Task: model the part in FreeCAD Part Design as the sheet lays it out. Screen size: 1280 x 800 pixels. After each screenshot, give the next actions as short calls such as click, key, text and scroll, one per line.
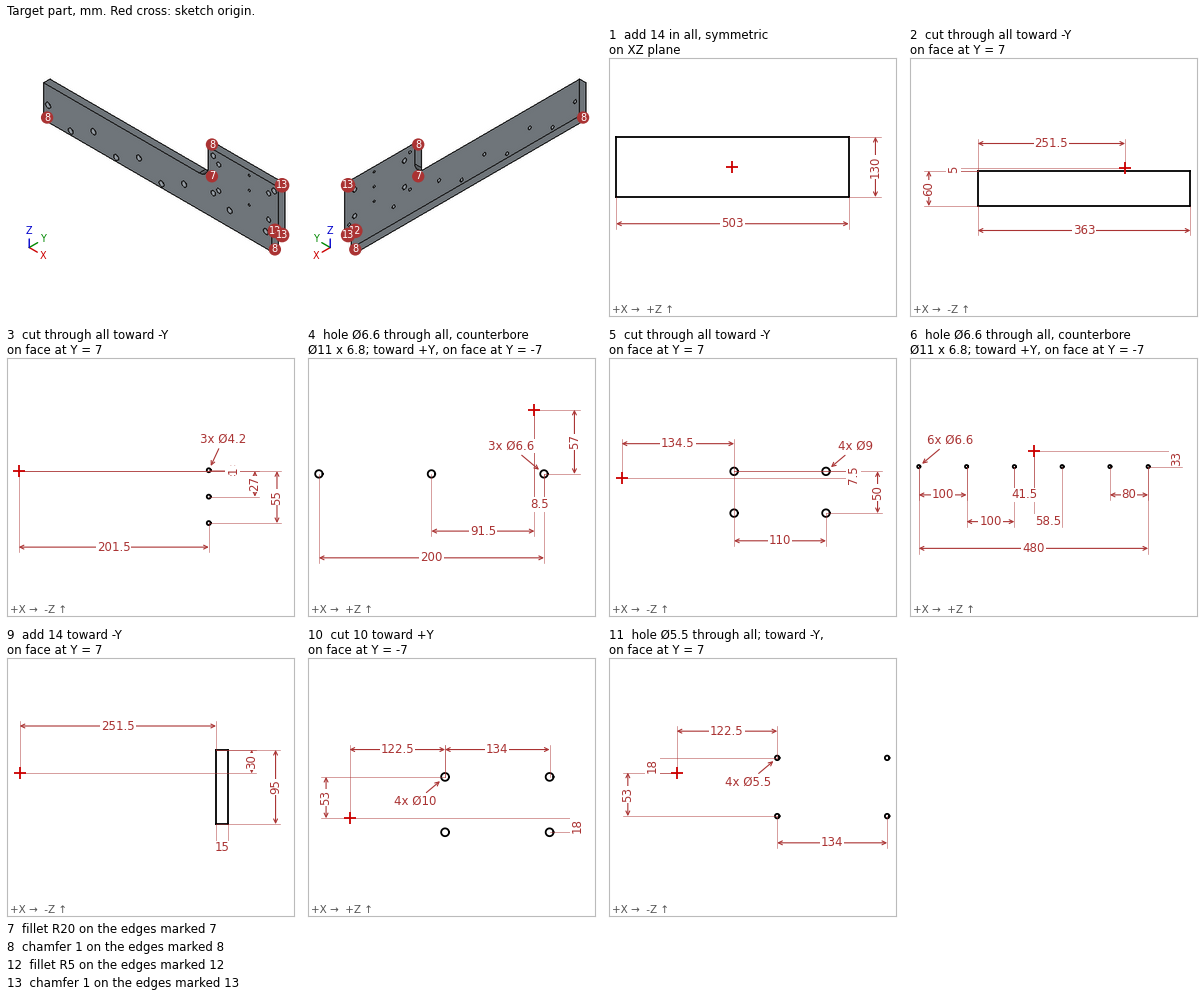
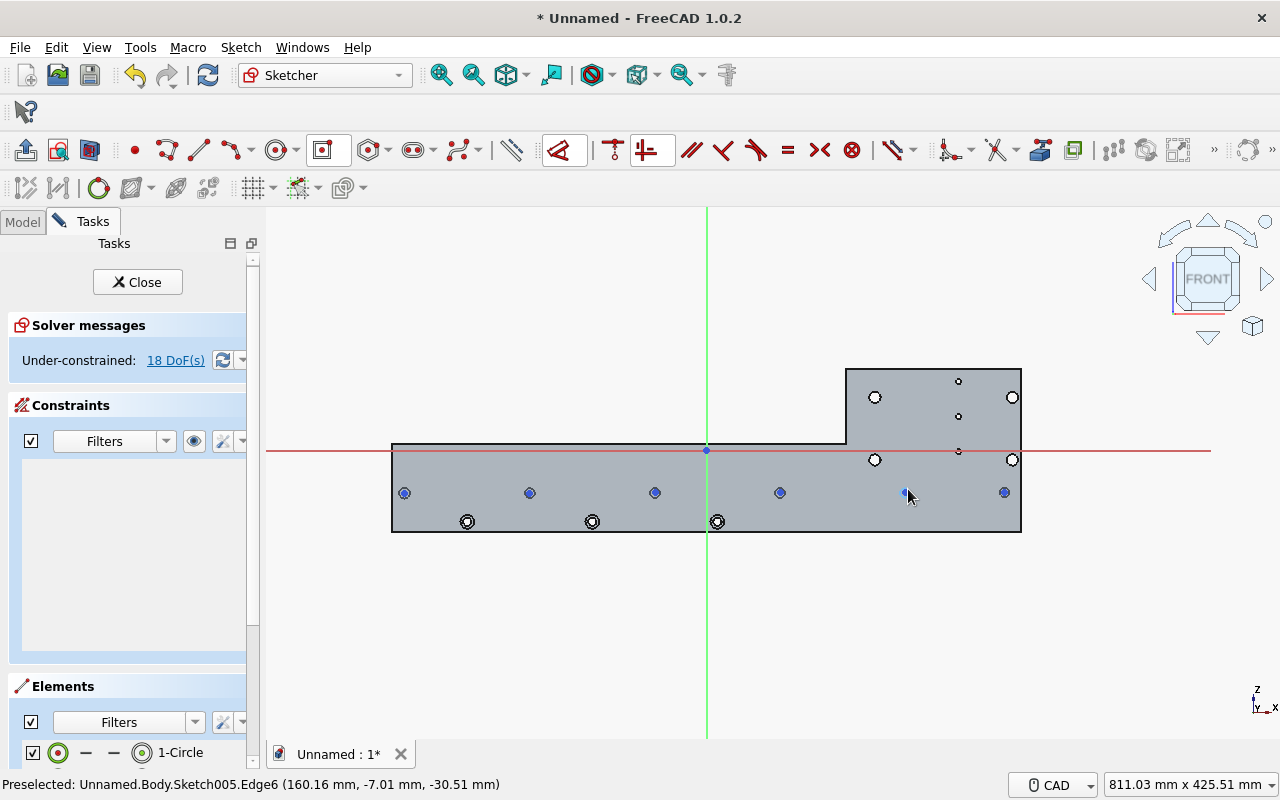
scroll(1008, 489, up, 6)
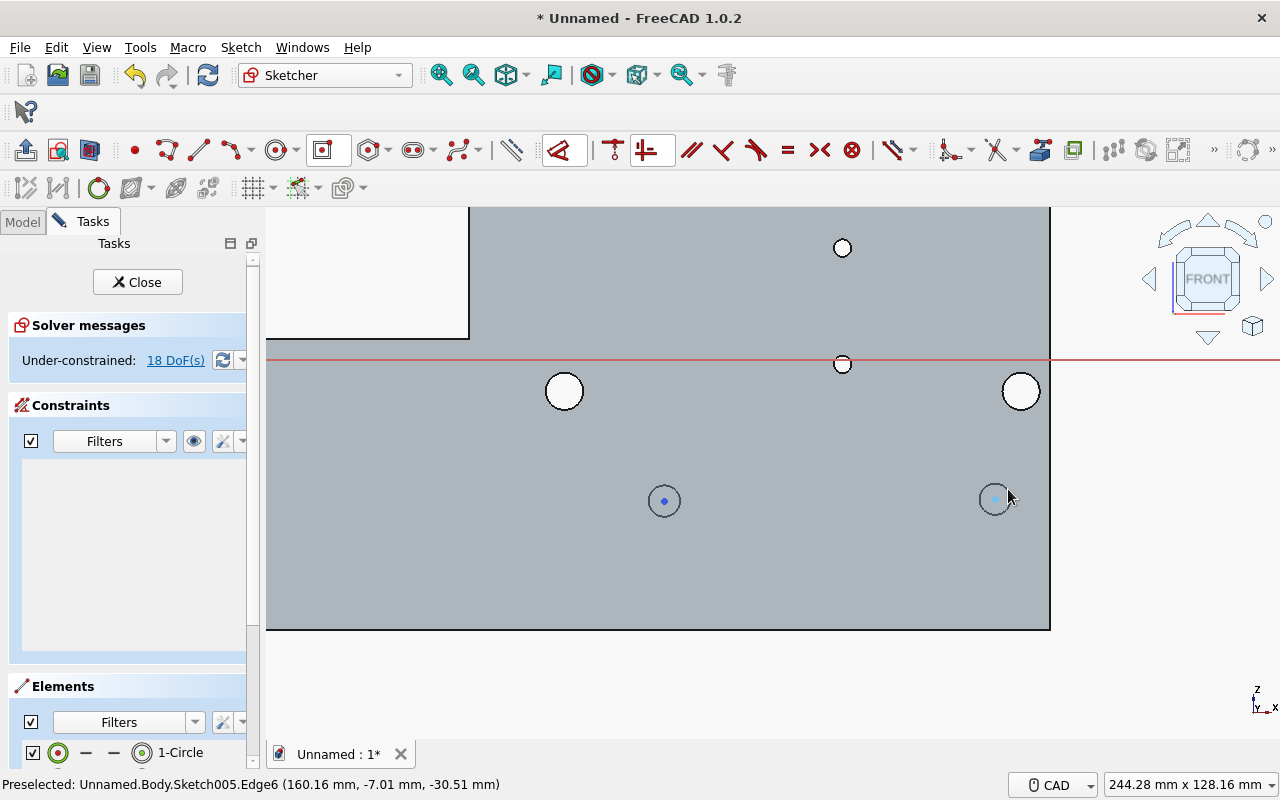
click(1006, 488)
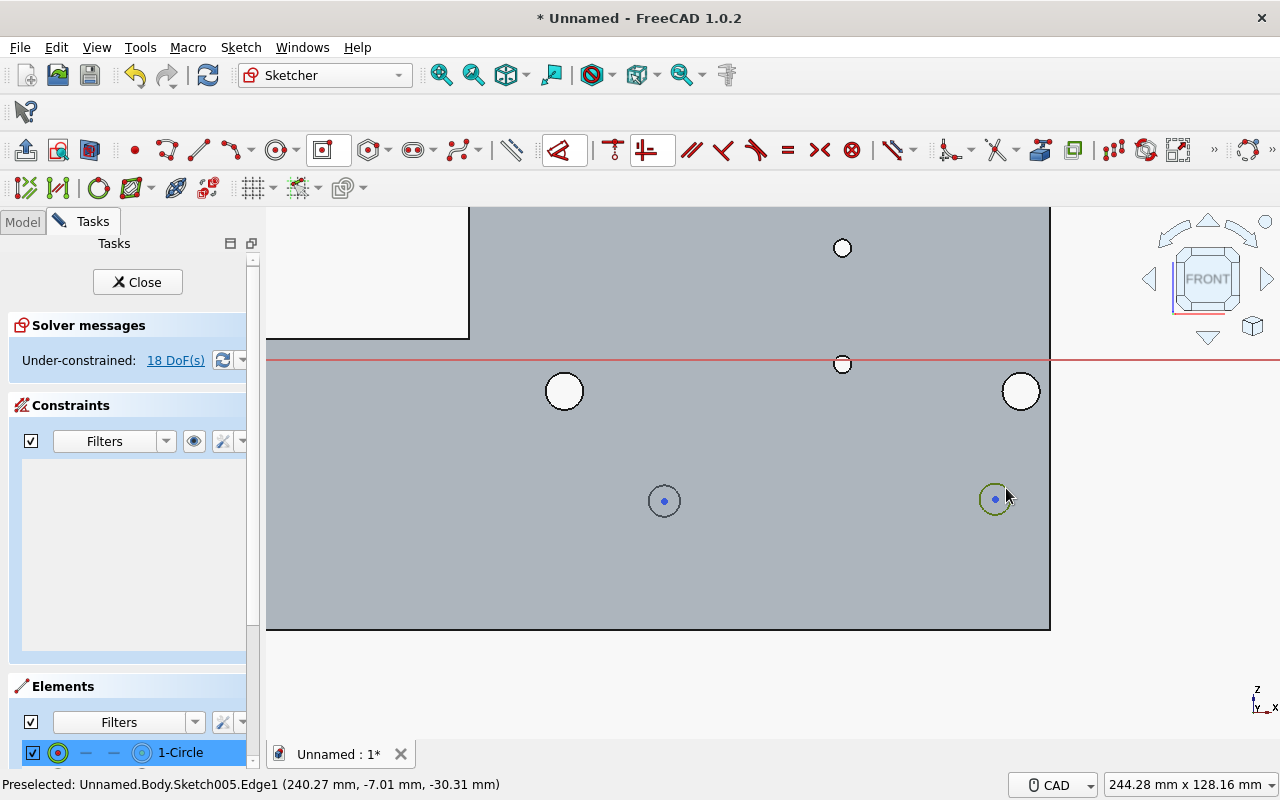
scroll(1008, 489, down, 6)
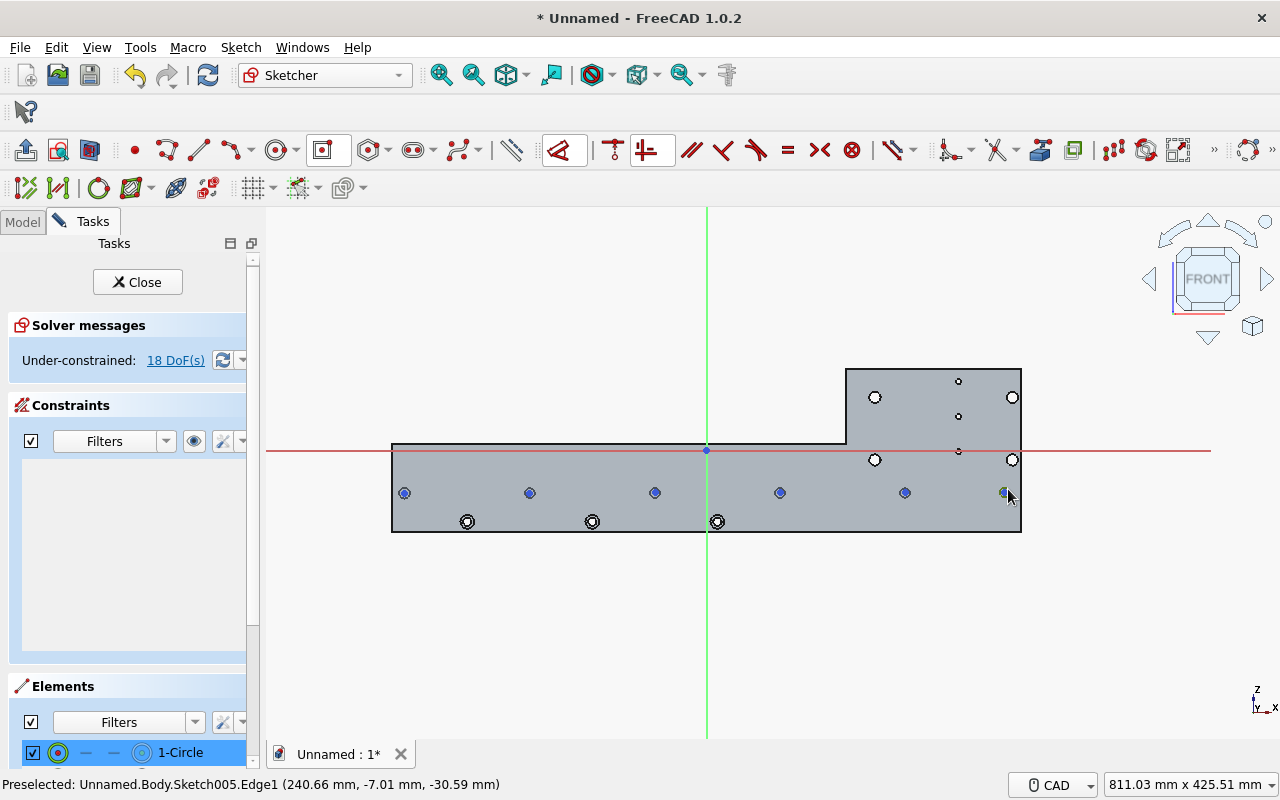
scroll(408, 489, up, 5)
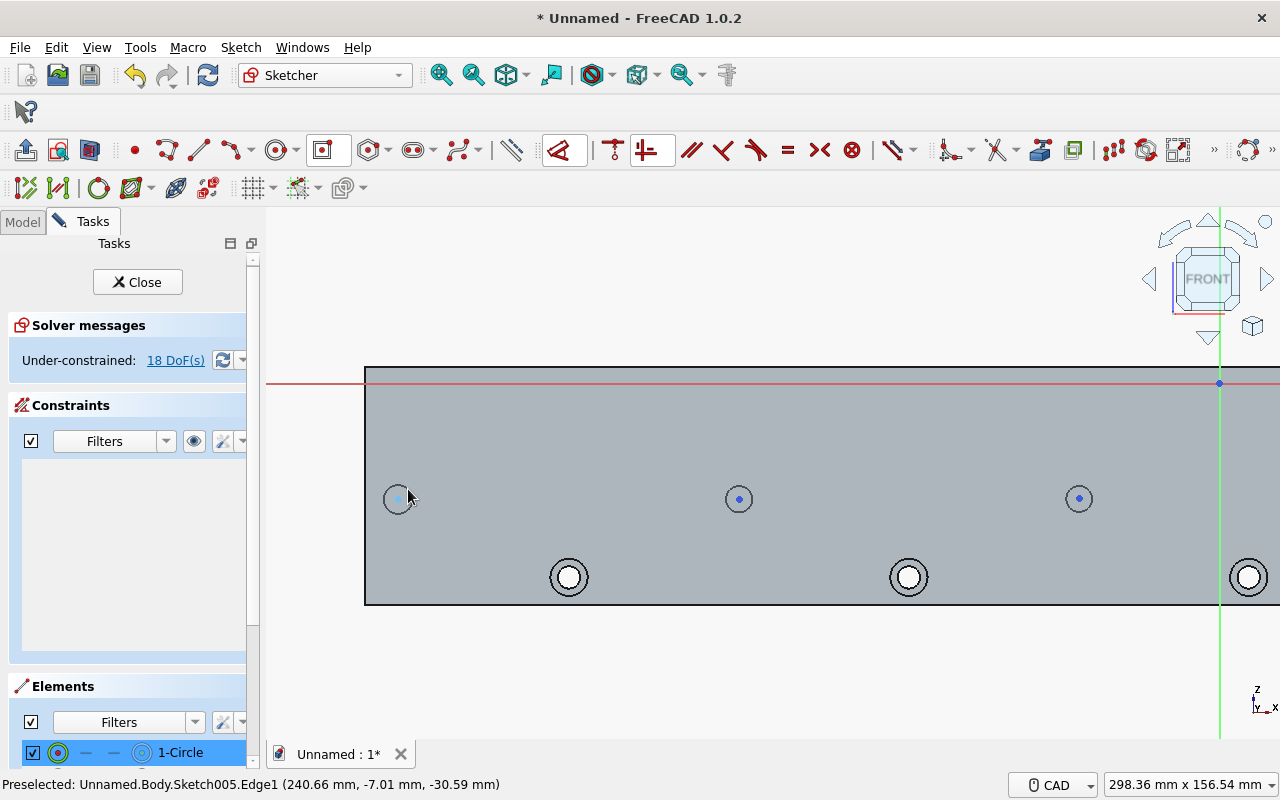
click(408, 489)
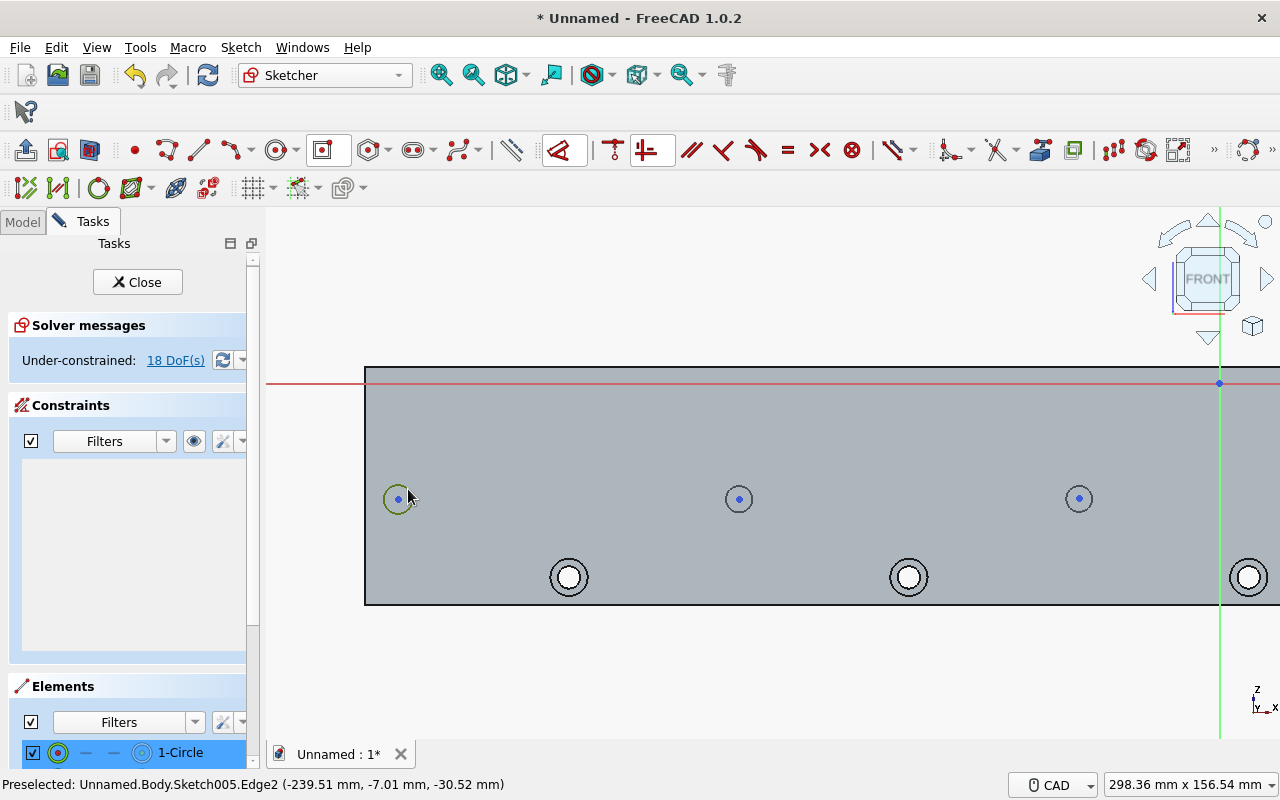
click(748, 490)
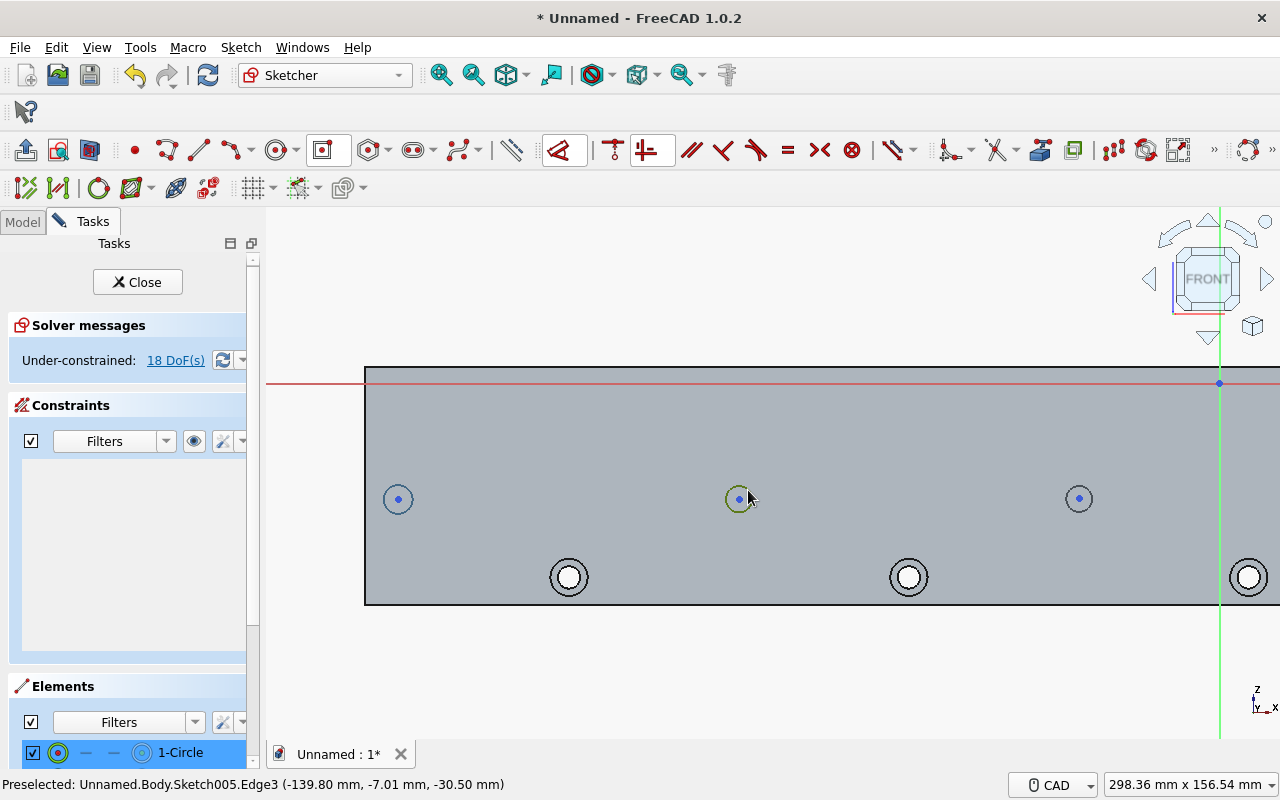
click(1088, 490)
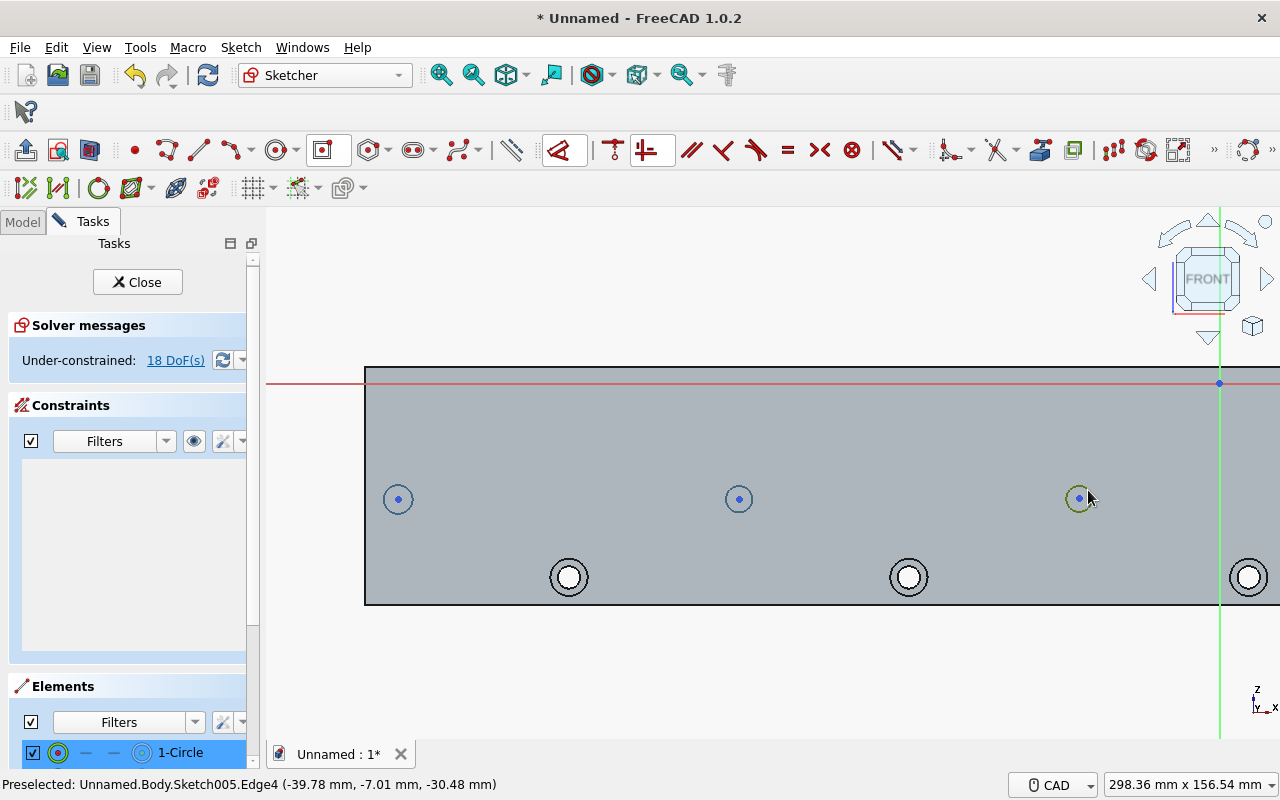
scroll(408, 489, down, 5)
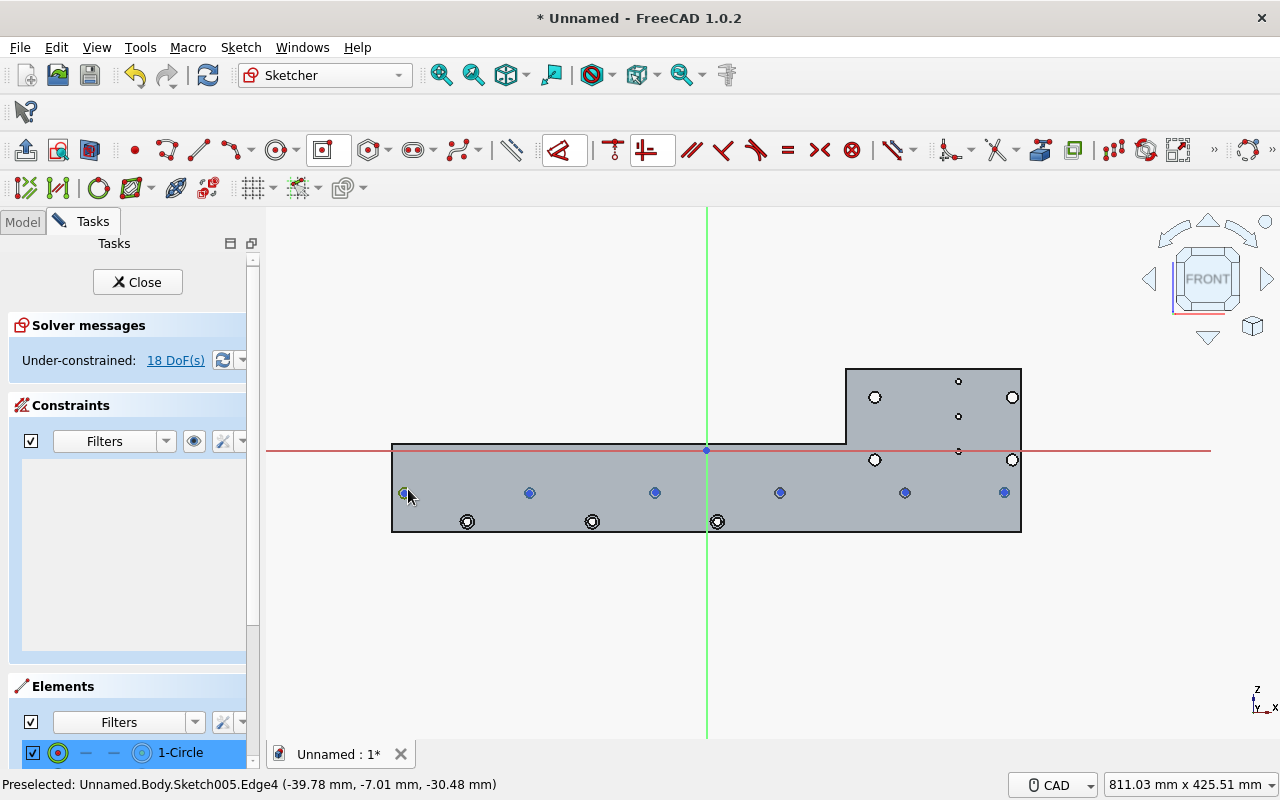
scroll(783, 490, up, 6)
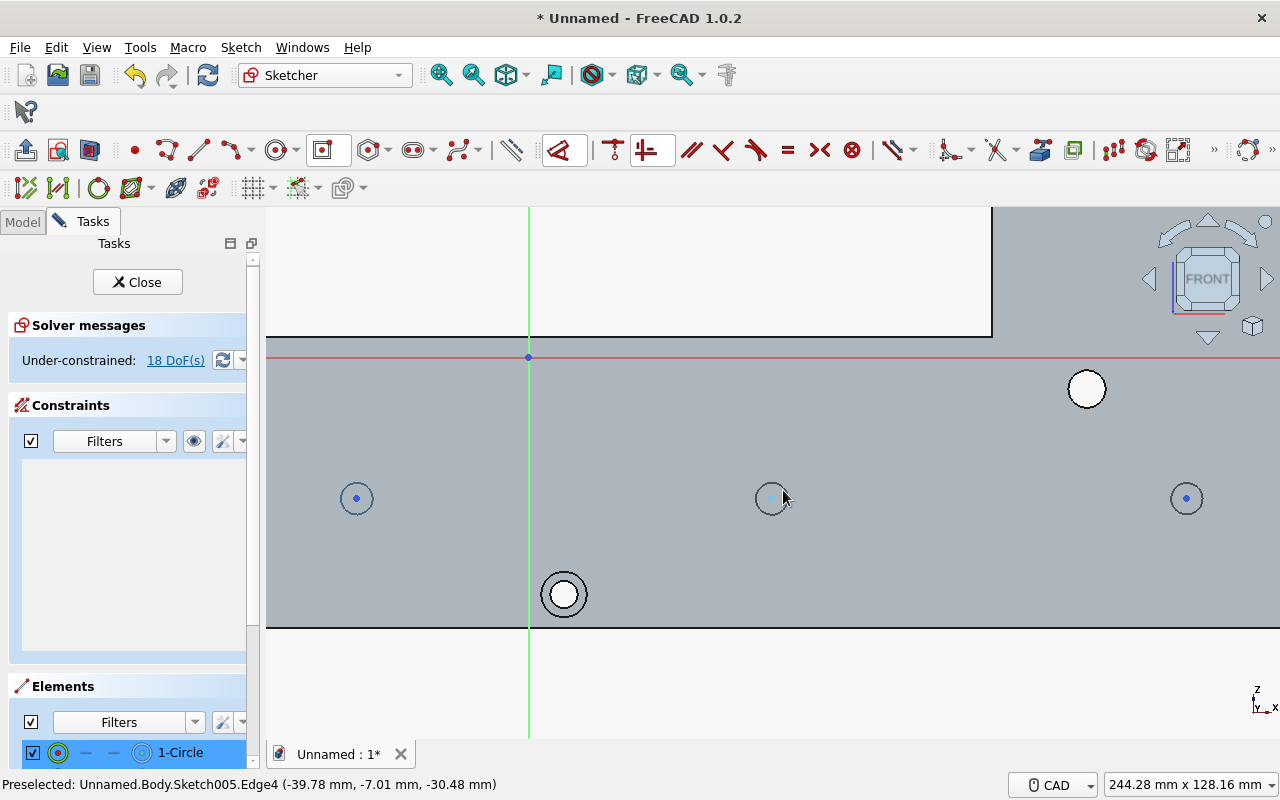
click(783, 487)